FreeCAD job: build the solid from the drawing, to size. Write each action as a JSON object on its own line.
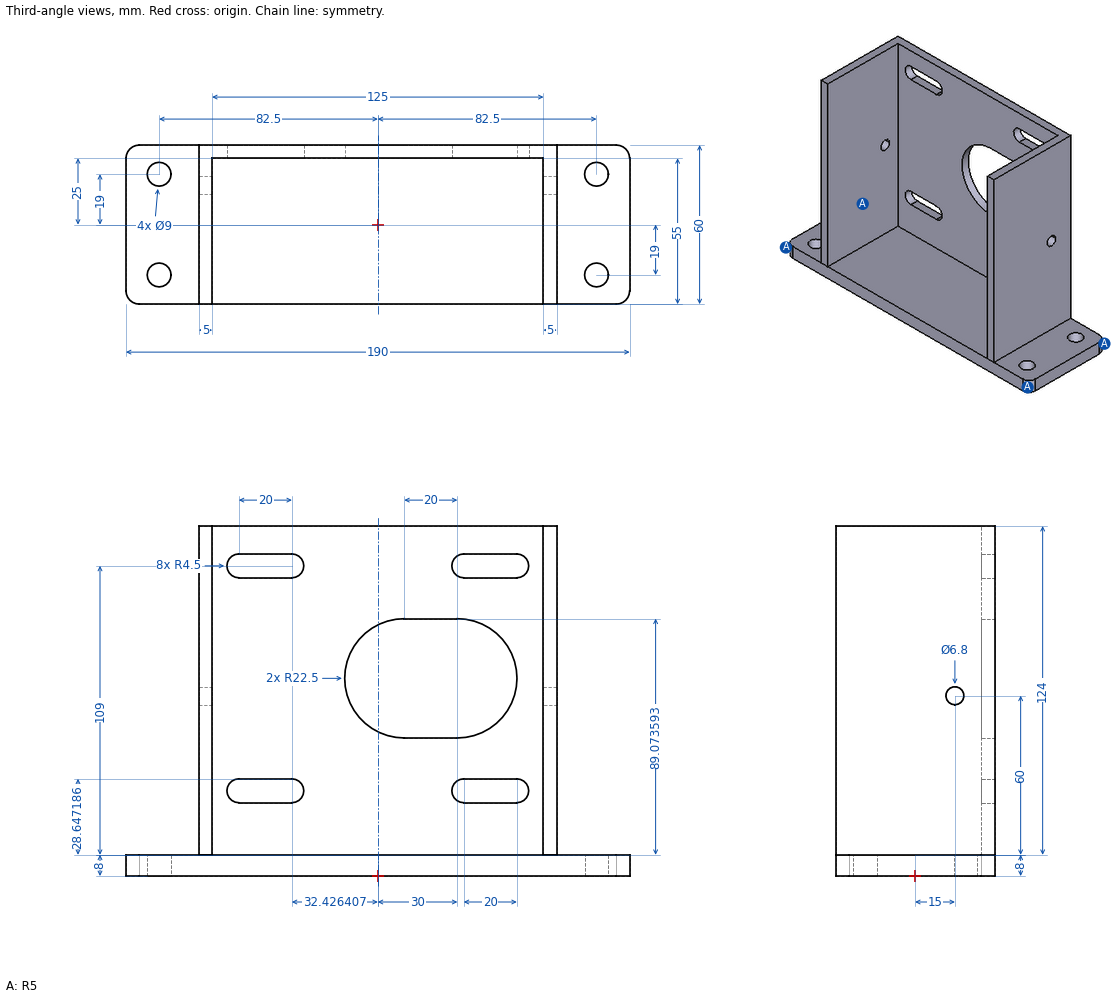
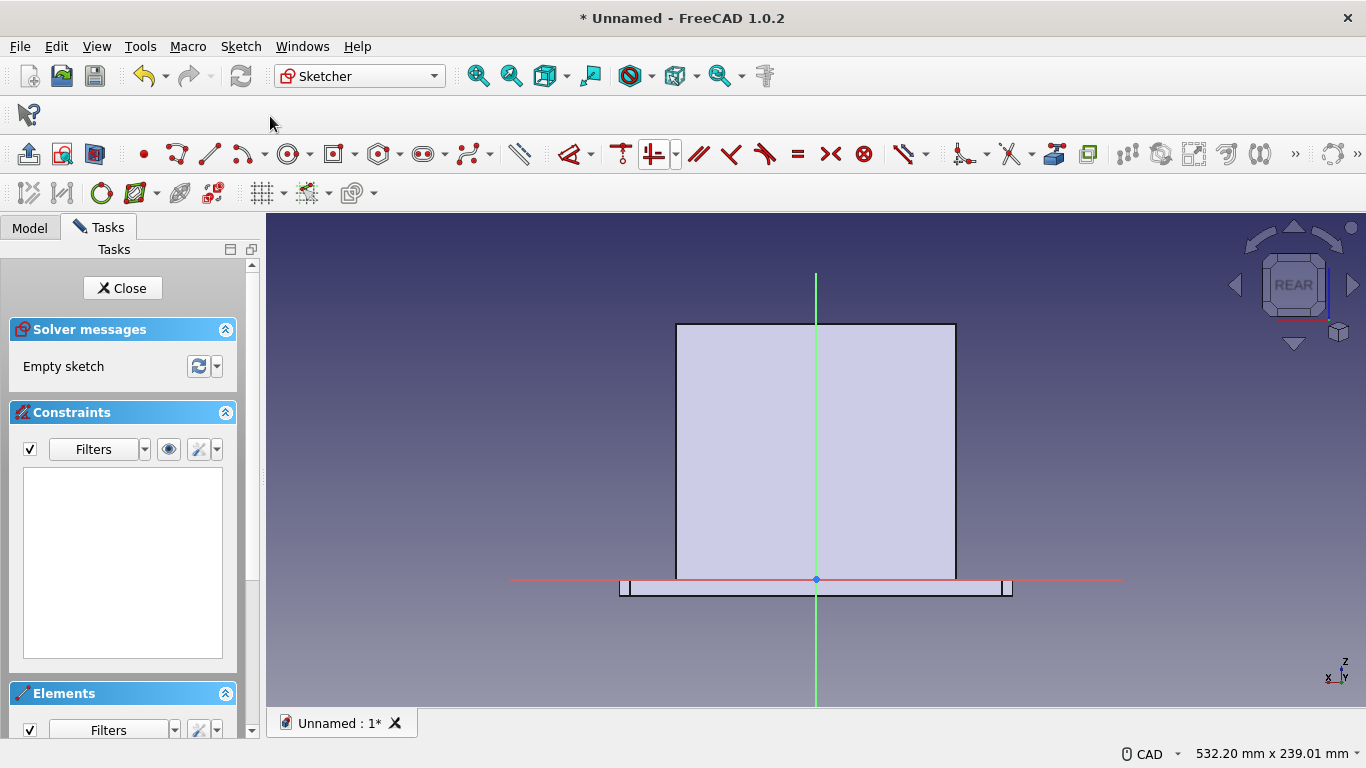
{"action": "left_click", "coordinate": [422, 154]}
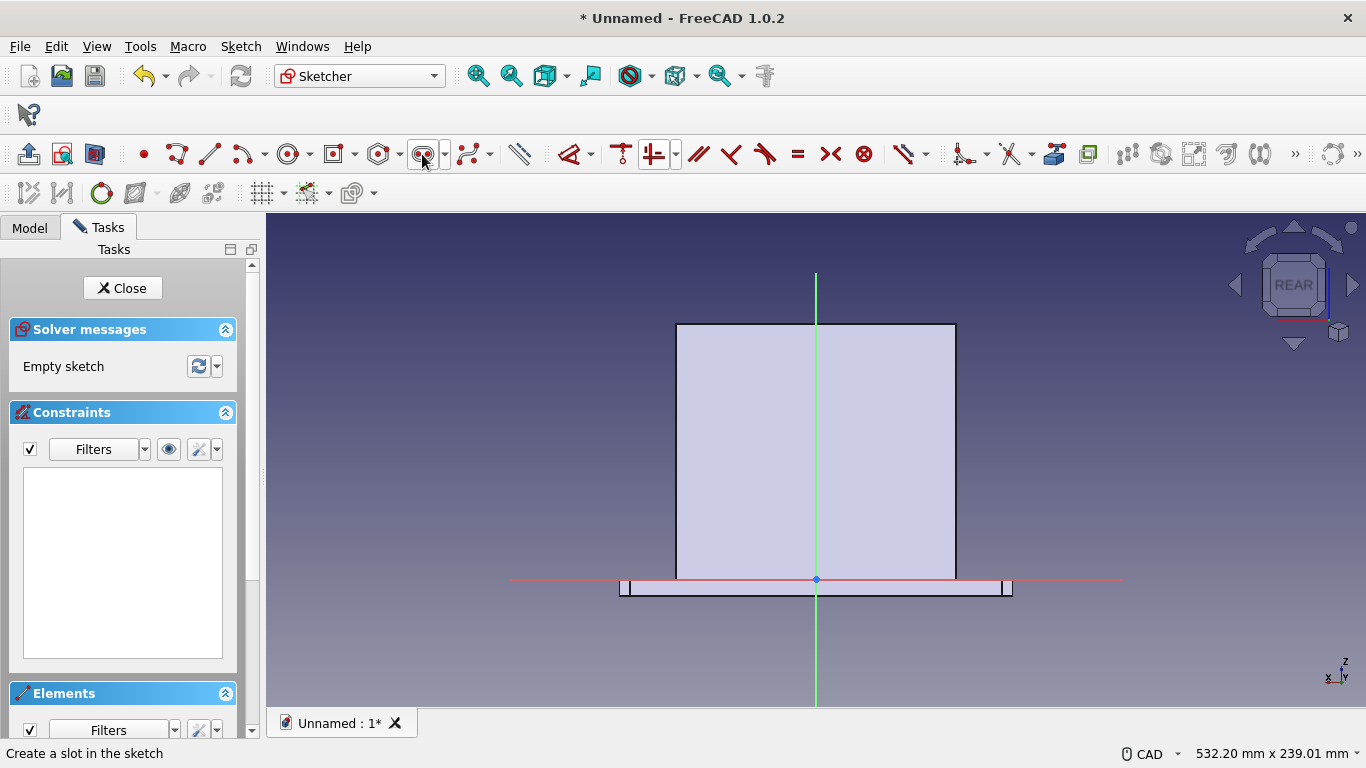
{"action": "scroll", "coordinate": [883, 355], "scroll_direction": "up", "scroll_amount": 5}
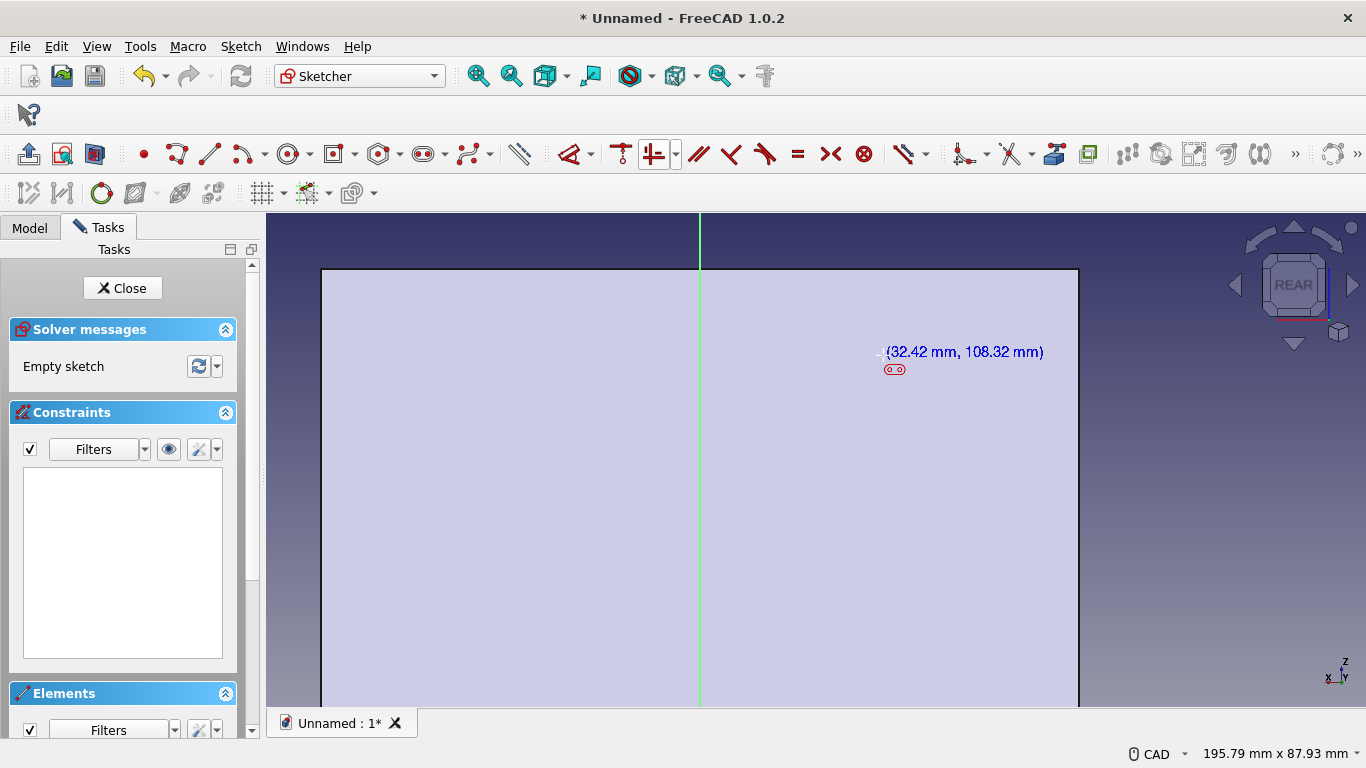
{"action": "left_click", "coordinate": [882, 353]}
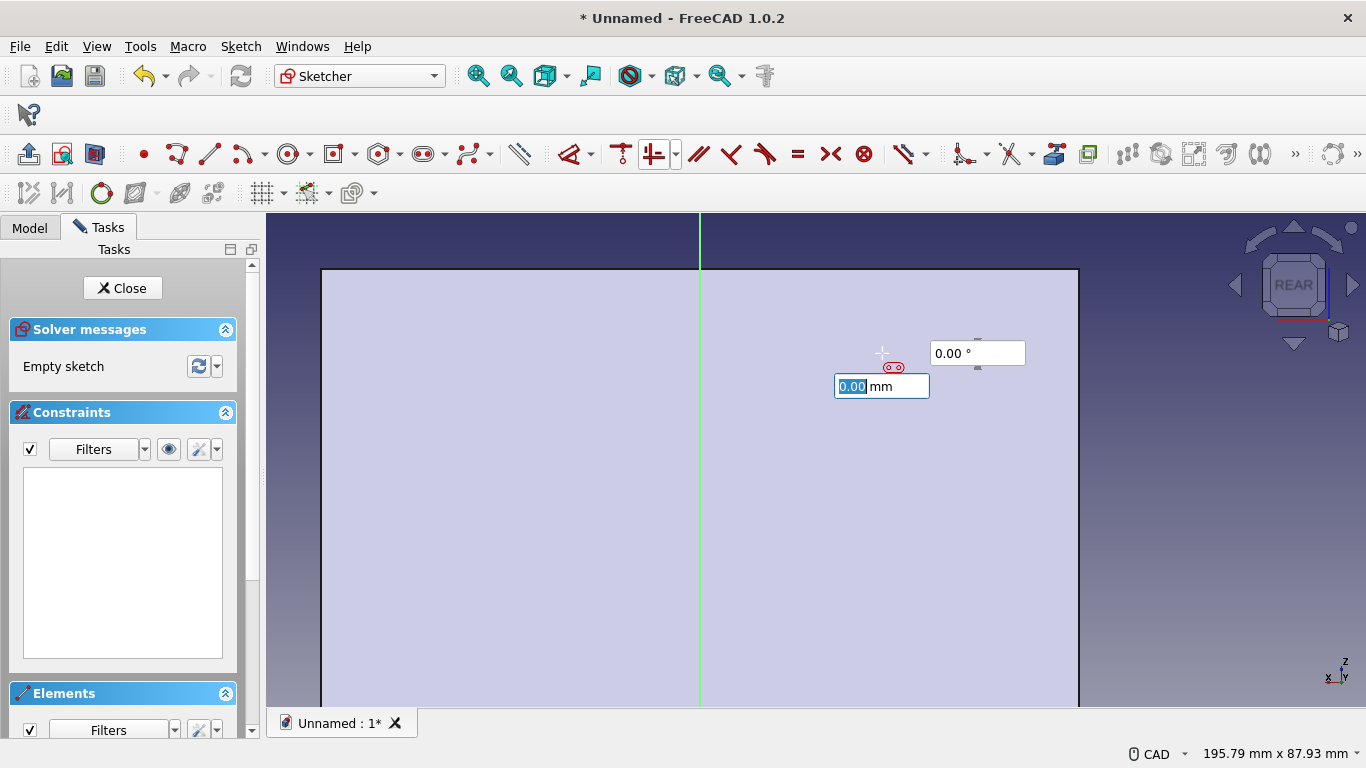
{"action": "left_click", "coordinate": [994, 353]}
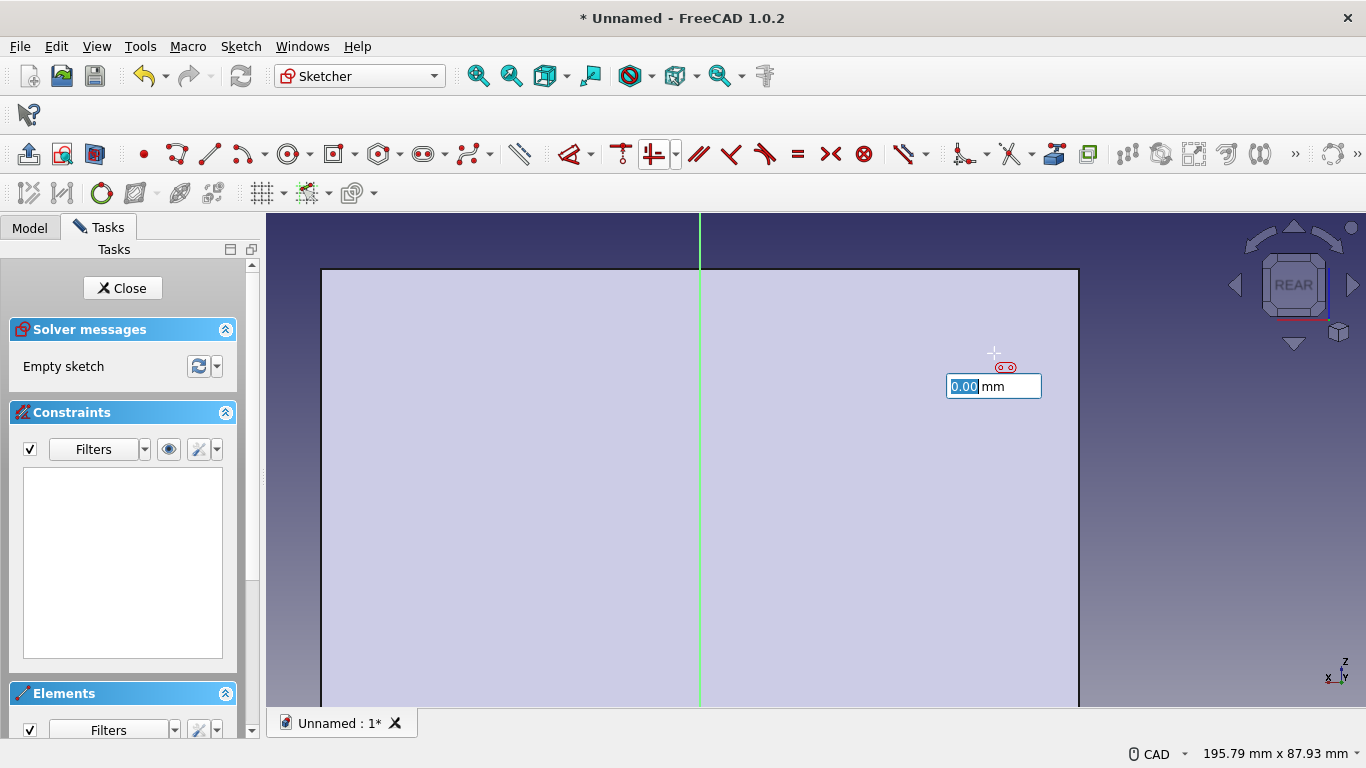
{"action": "left_click", "coordinate": [938, 379]}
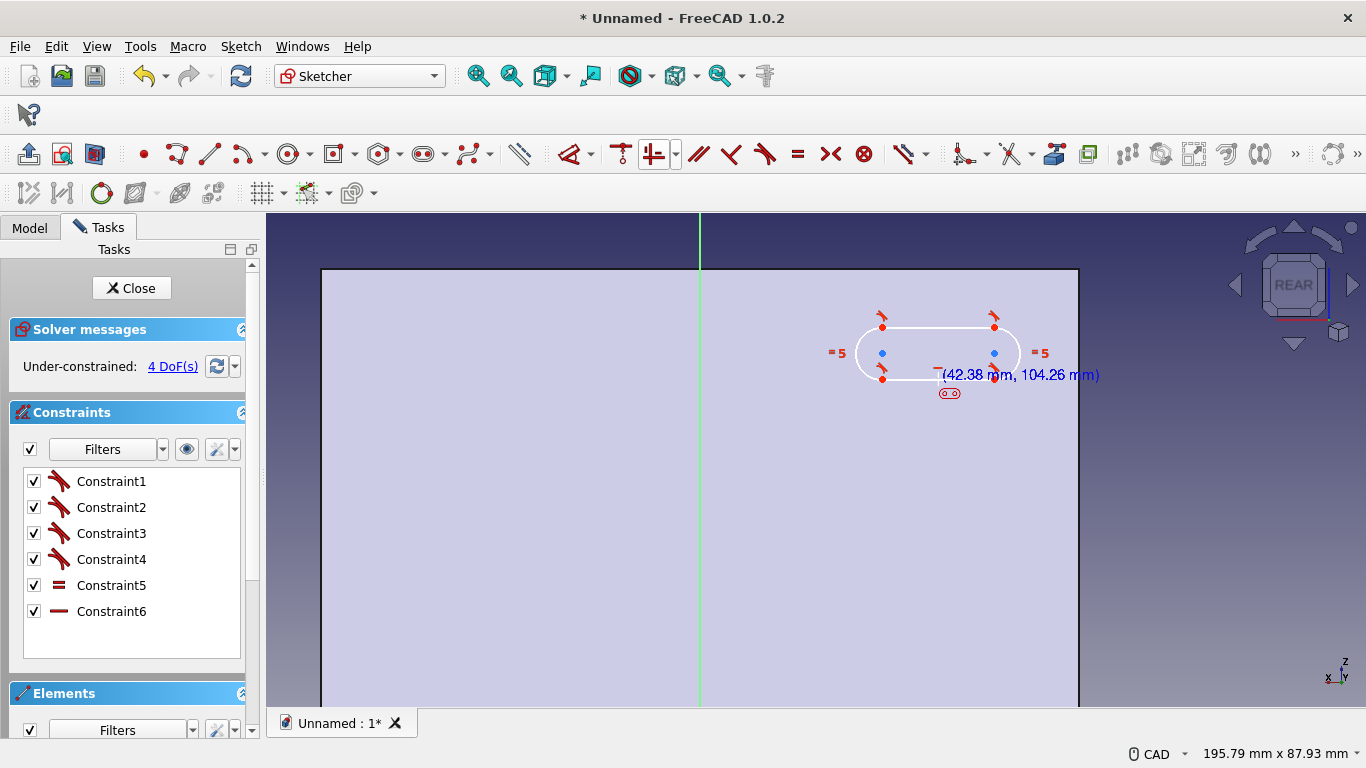
{"action": "scroll", "coordinate": [786, 307], "scroll_direction": "down", "scroll_amount": 4}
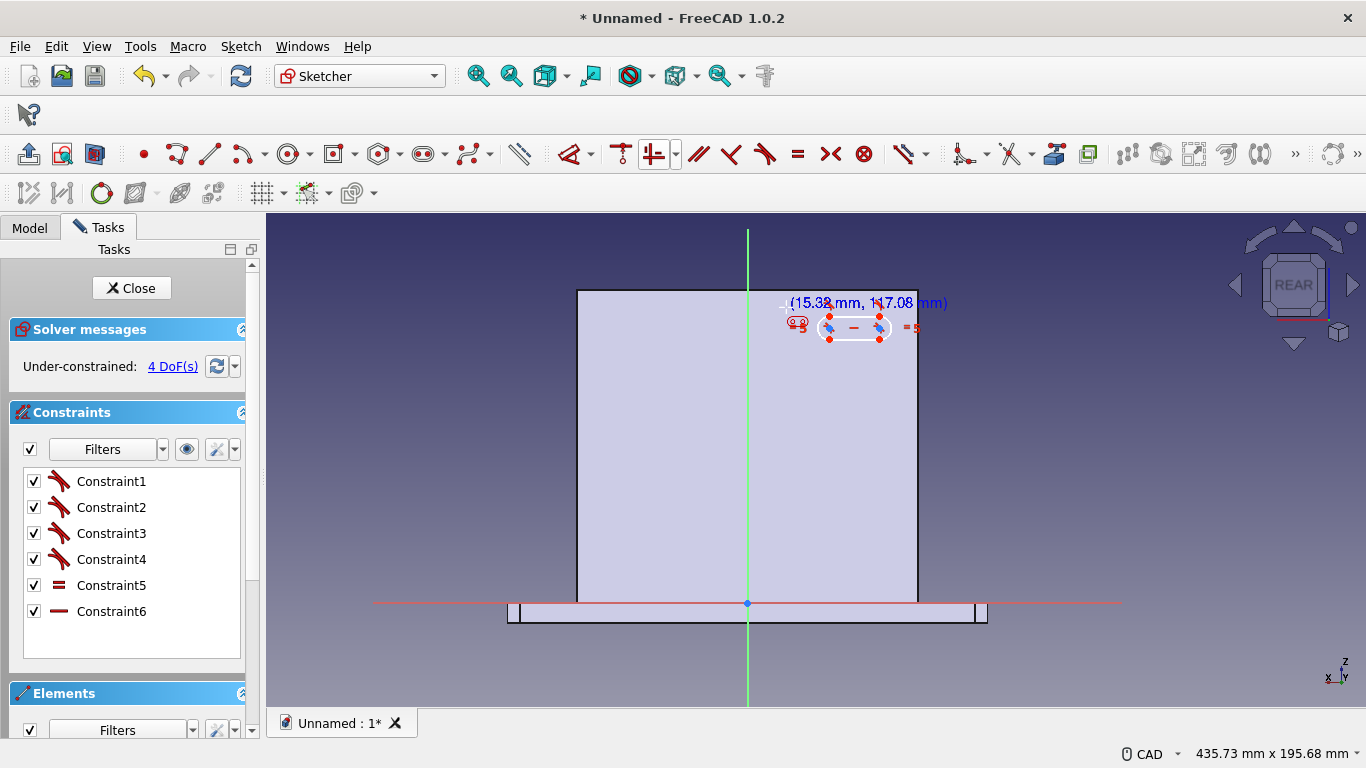
{"action": "scroll", "coordinate": [829, 542], "scroll_direction": "up", "scroll_amount": 4}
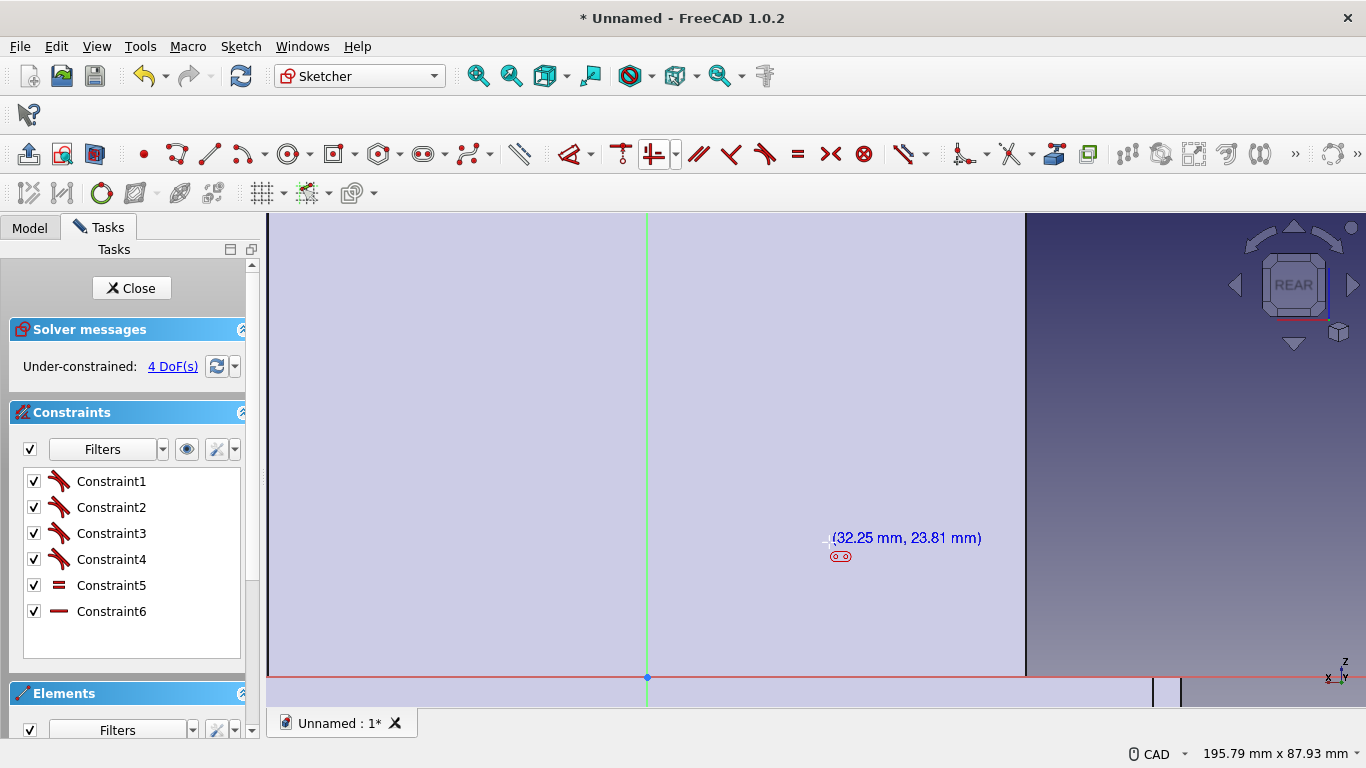
{"action": "left_click", "coordinate": [829, 542]}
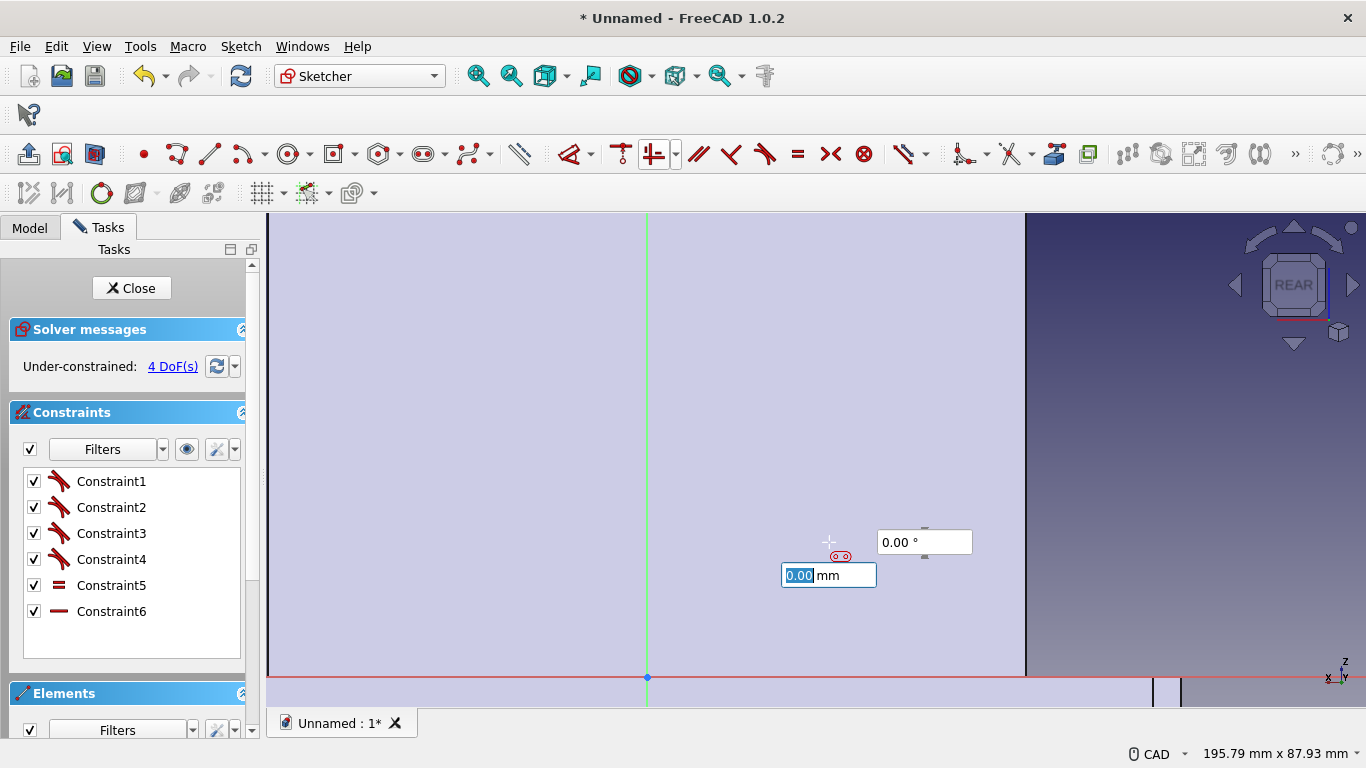
{"action": "left_click", "coordinate": [942, 542]}